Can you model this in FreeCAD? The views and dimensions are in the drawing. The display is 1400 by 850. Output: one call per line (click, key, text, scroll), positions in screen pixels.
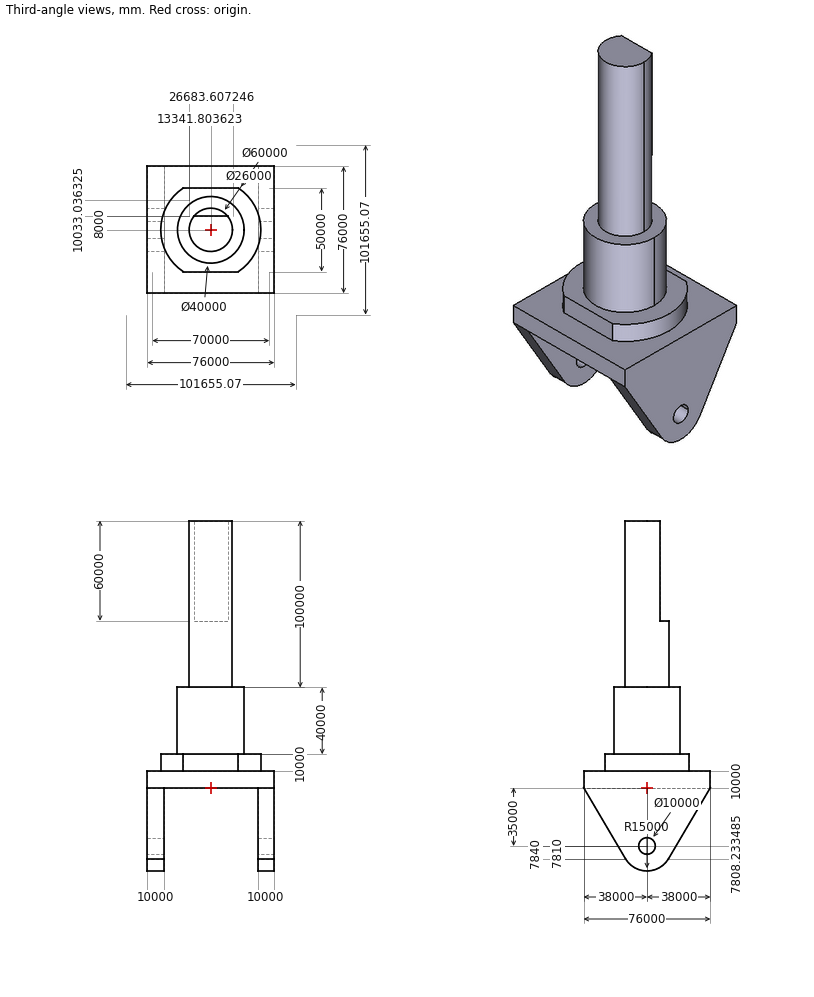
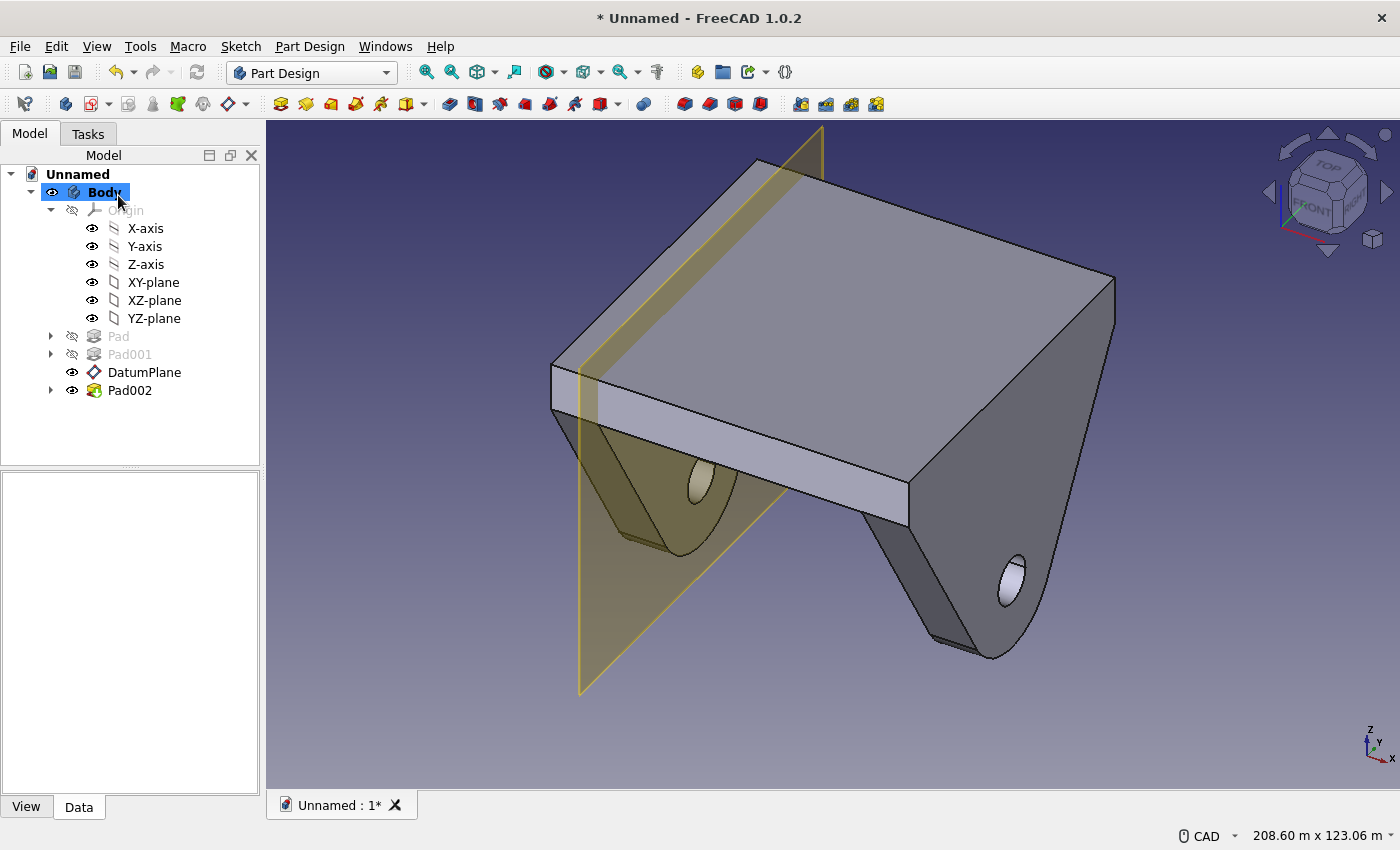
click(117, 372)
key(space)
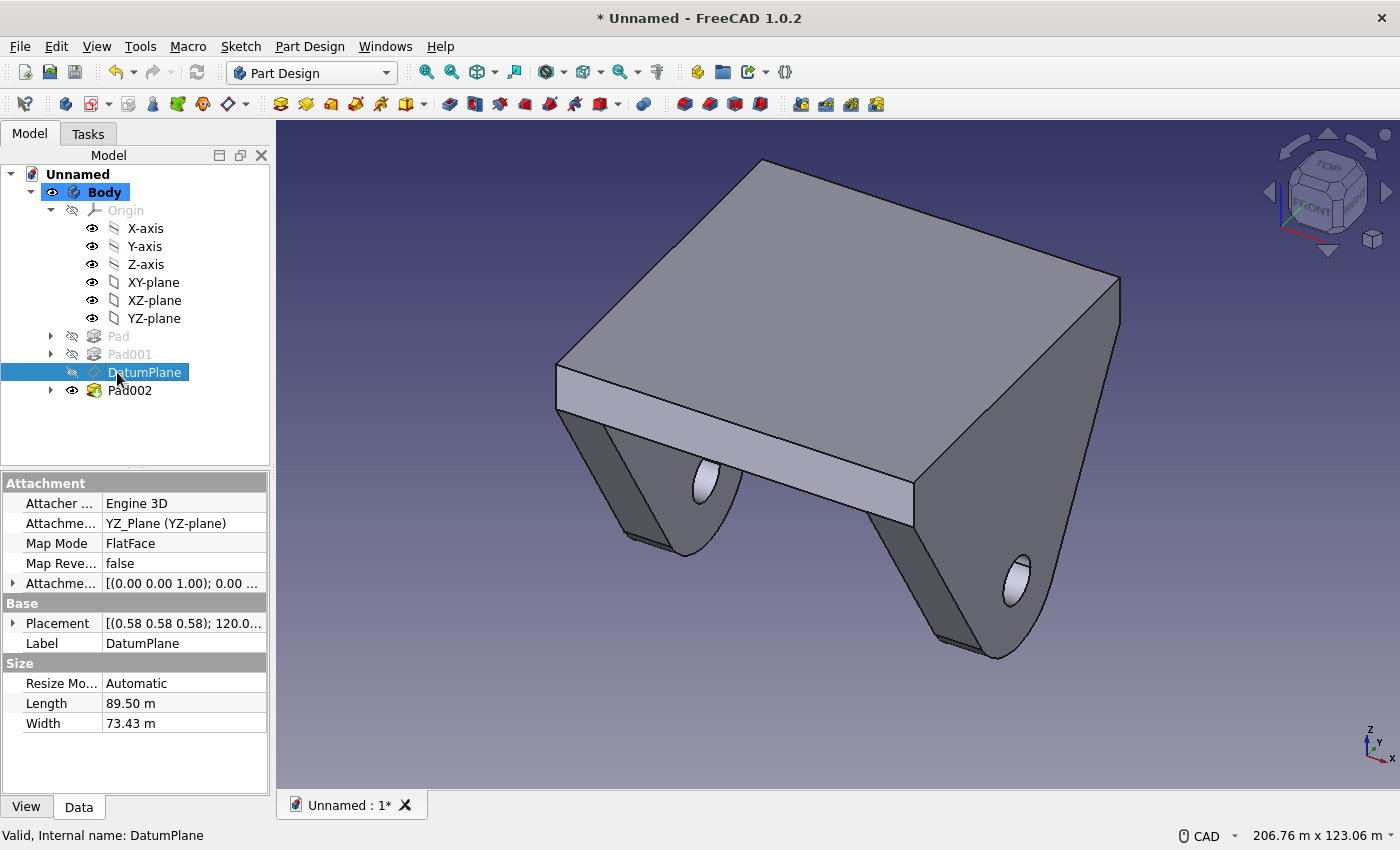
click(838, 320)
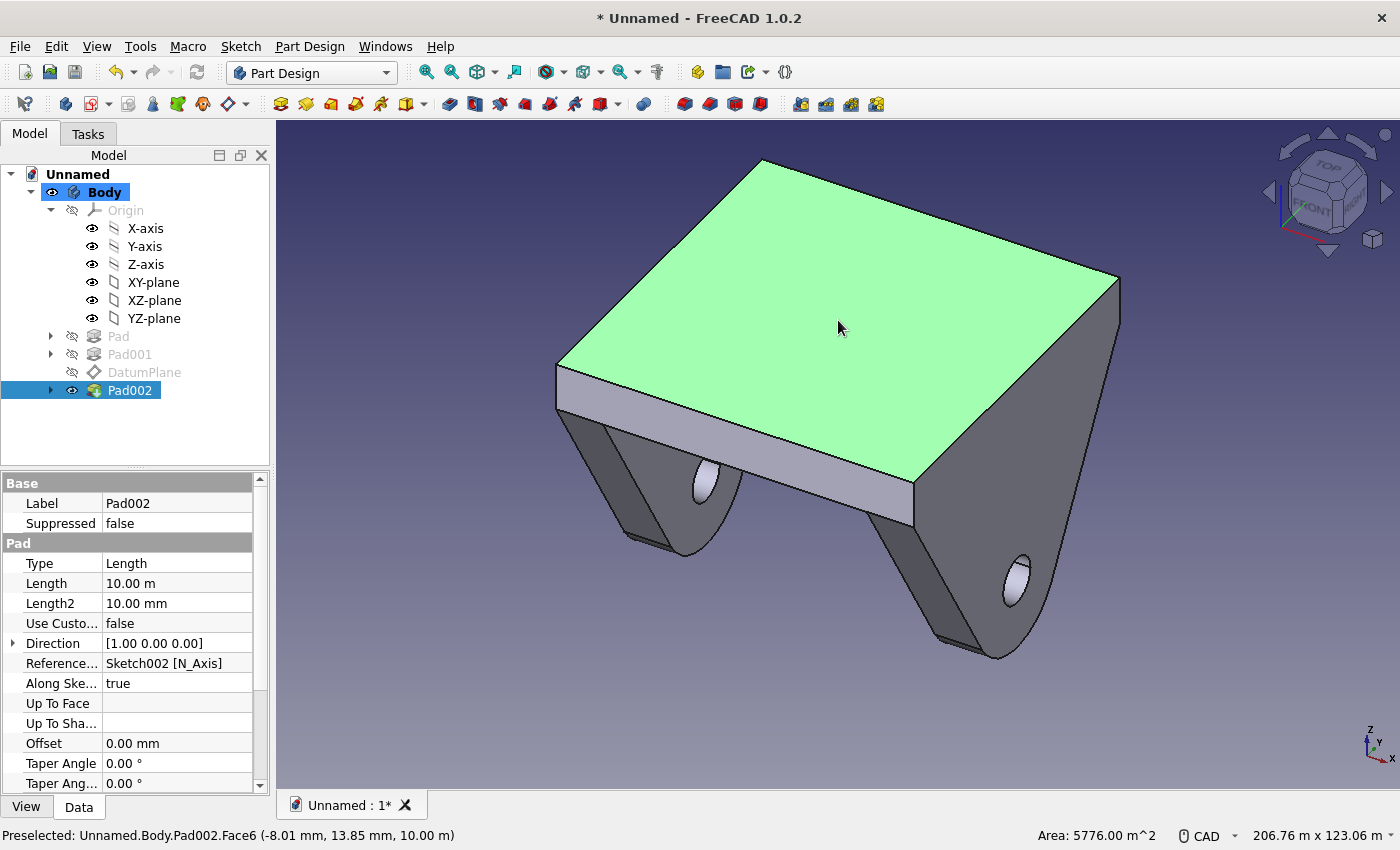
click(90, 104)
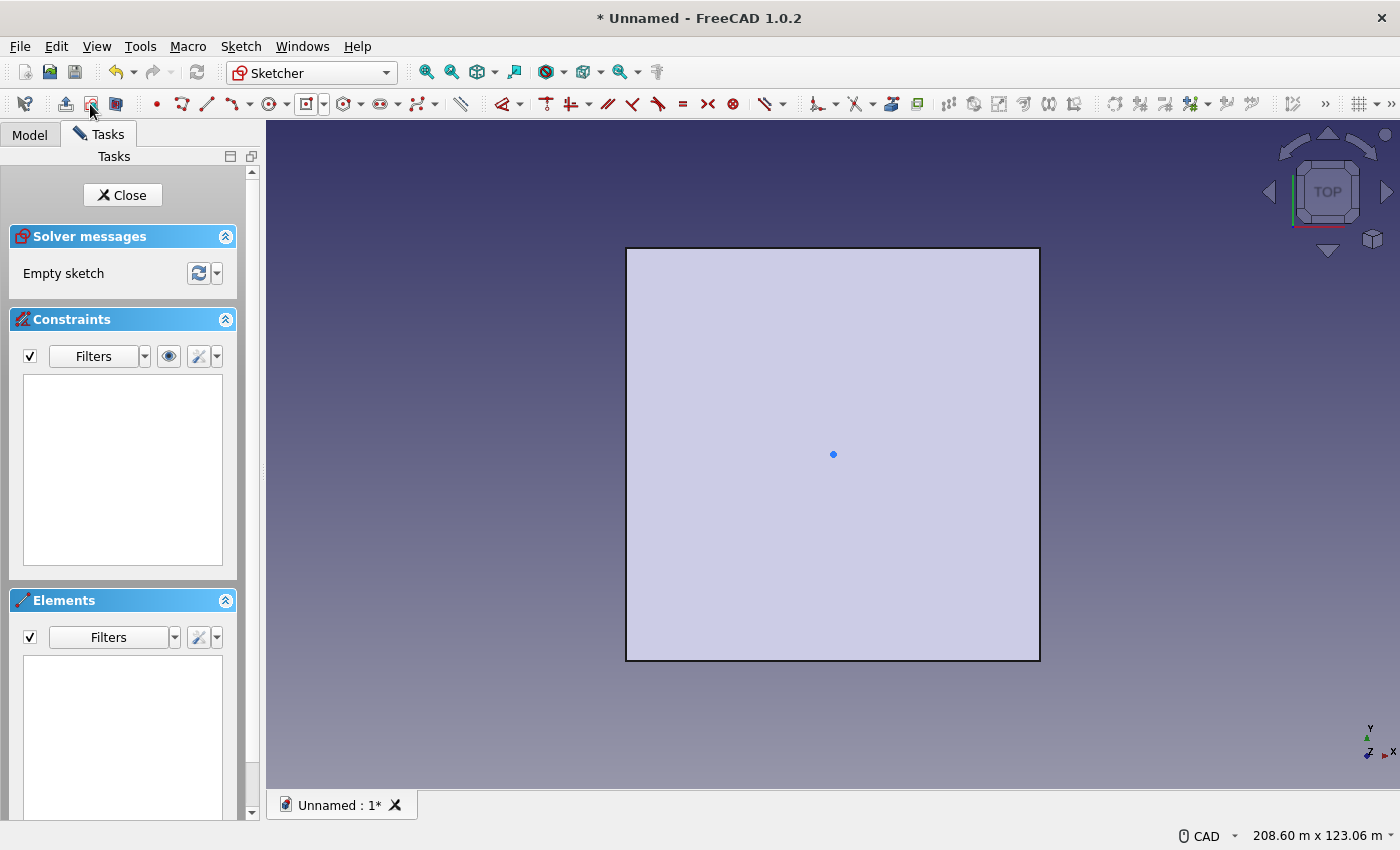
click(268, 104)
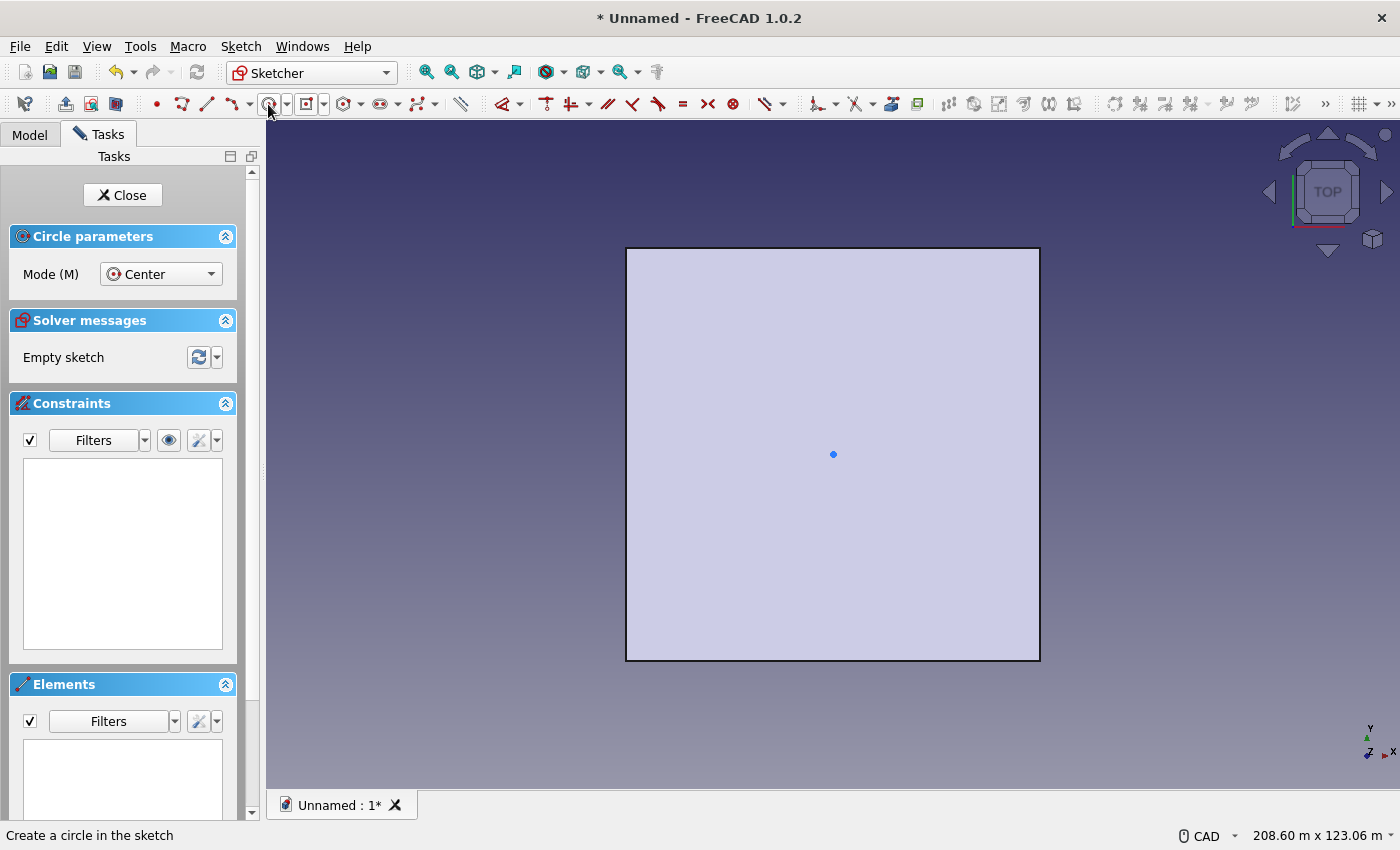
click(833, 455)
click(948, 339)
key(Escape)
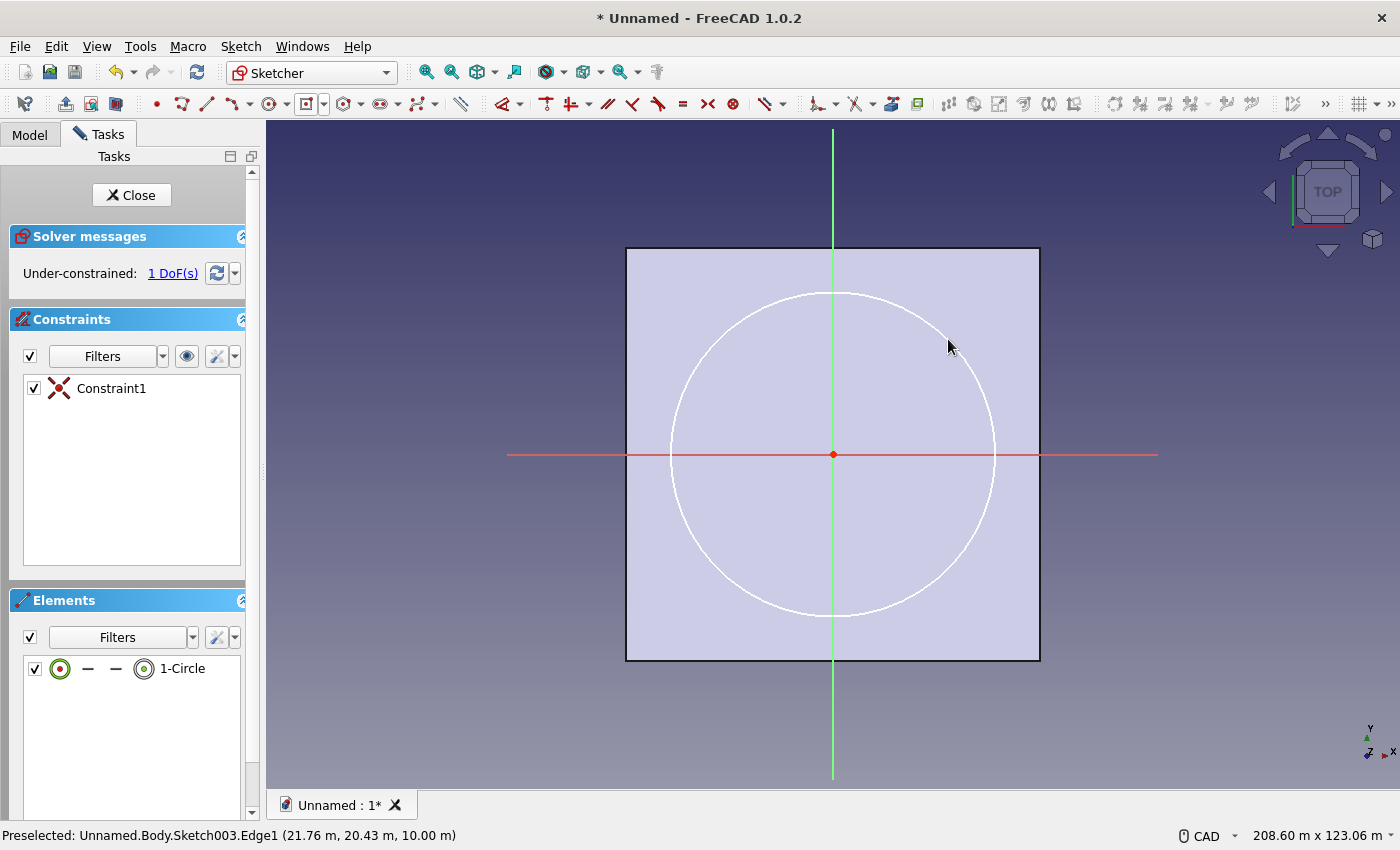
click(502, 104)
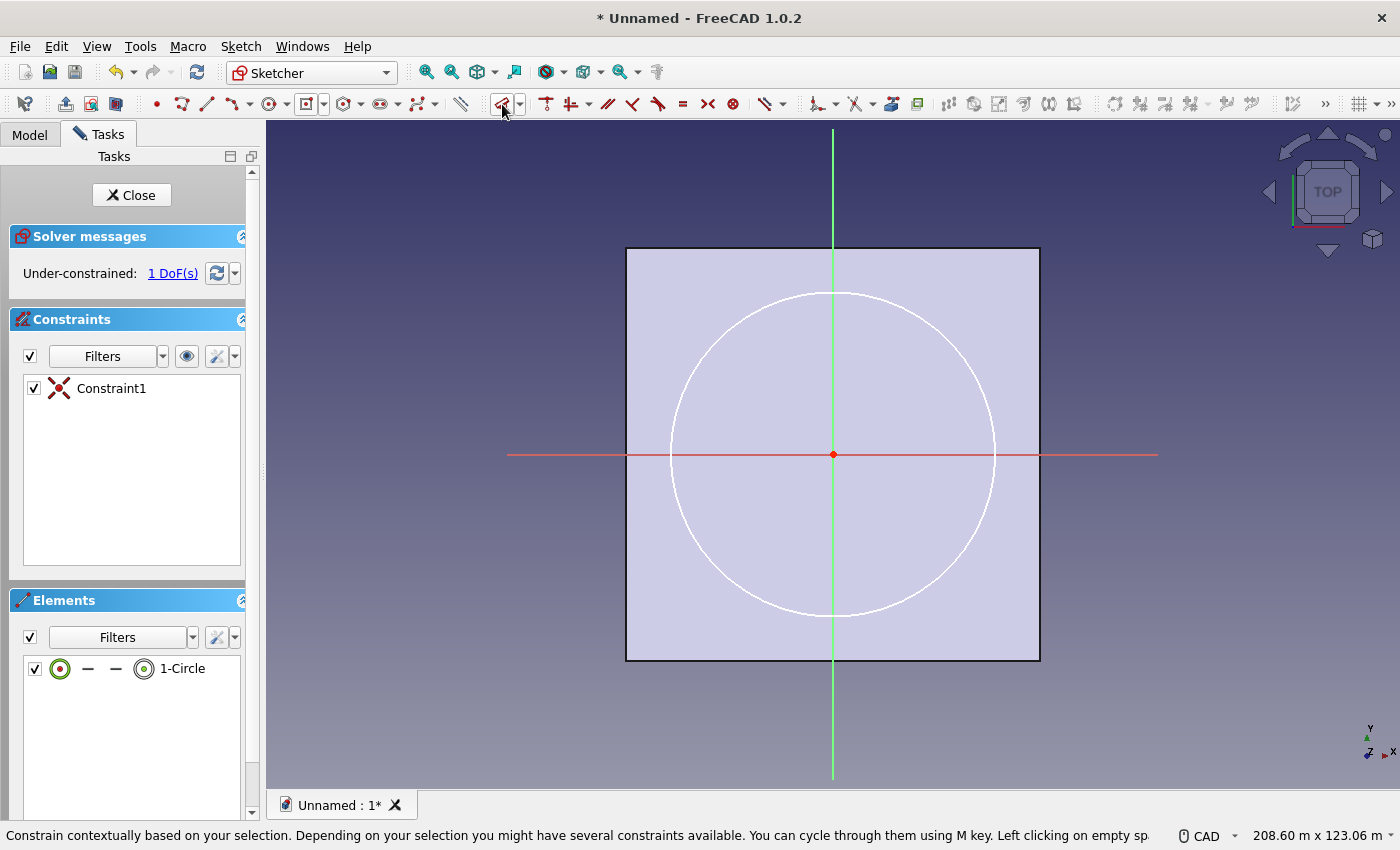
click(947, 339)
click(969, 316)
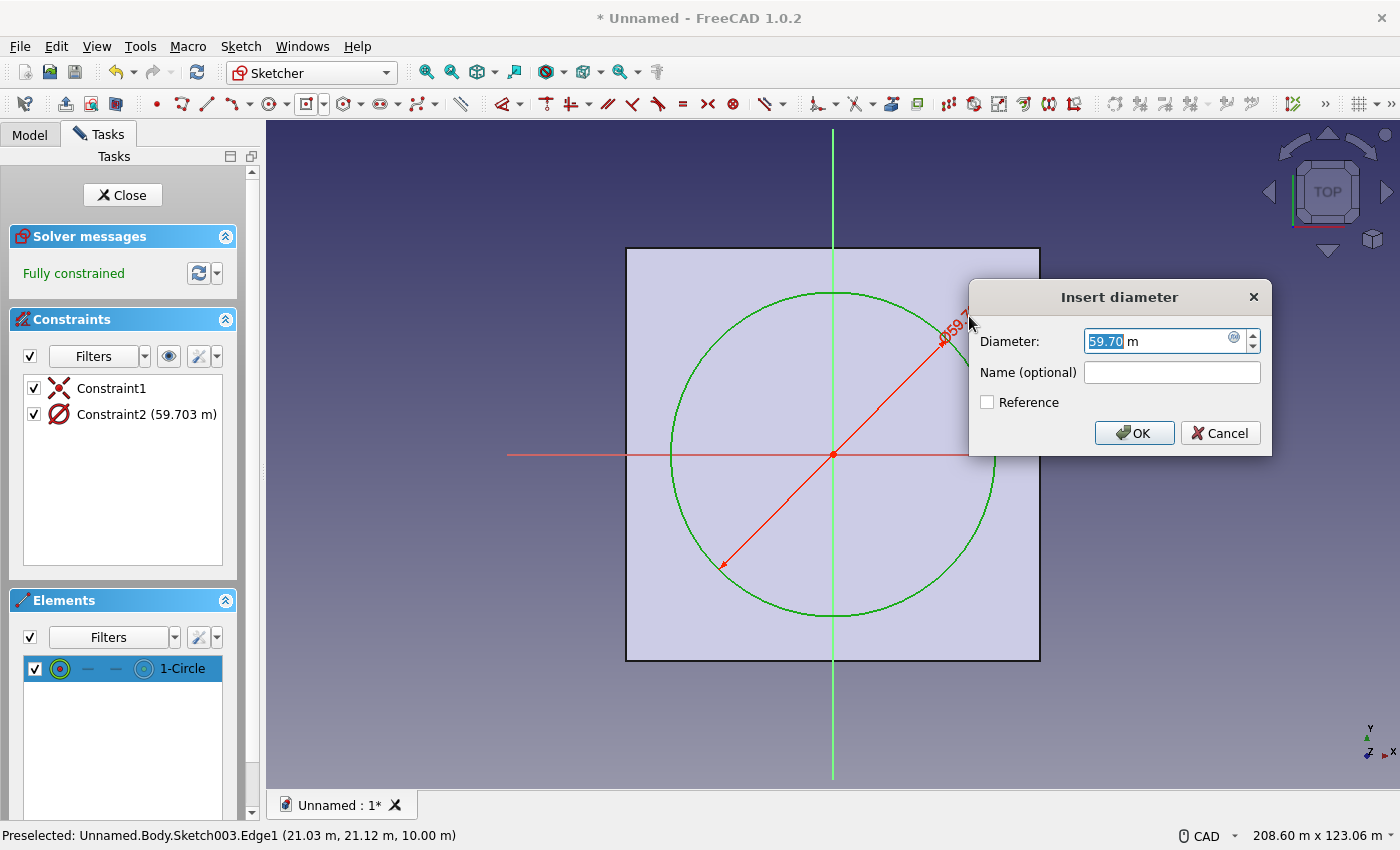
key(ctrl+a)
text(60000 mm)
key(Return)
key(Escape)